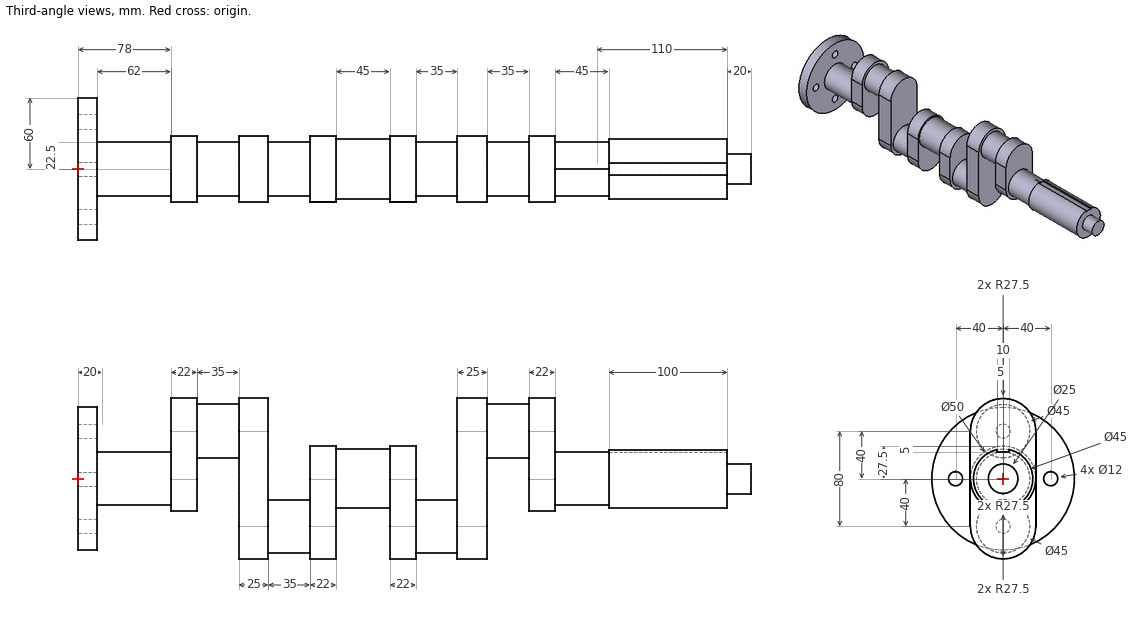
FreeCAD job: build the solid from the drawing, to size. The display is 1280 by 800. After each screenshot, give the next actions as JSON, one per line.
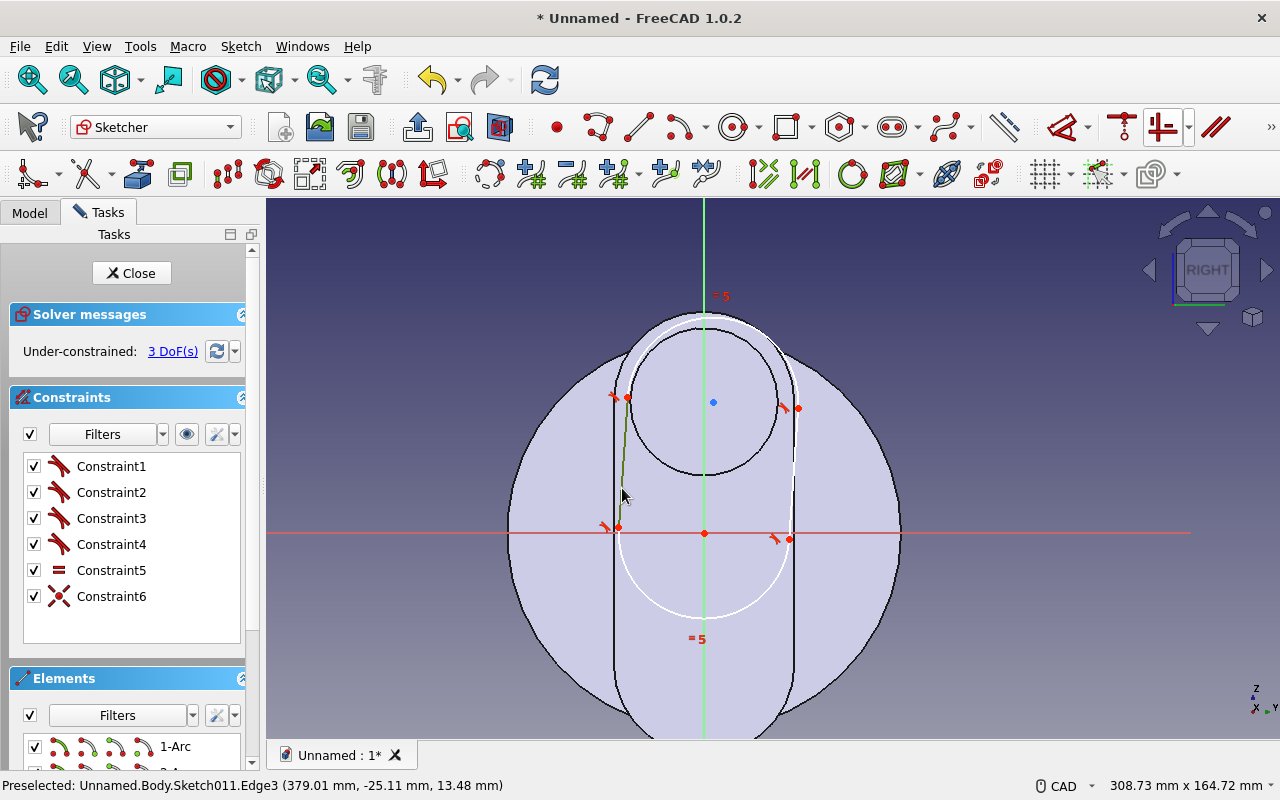
{"action": "key", "text": "v"}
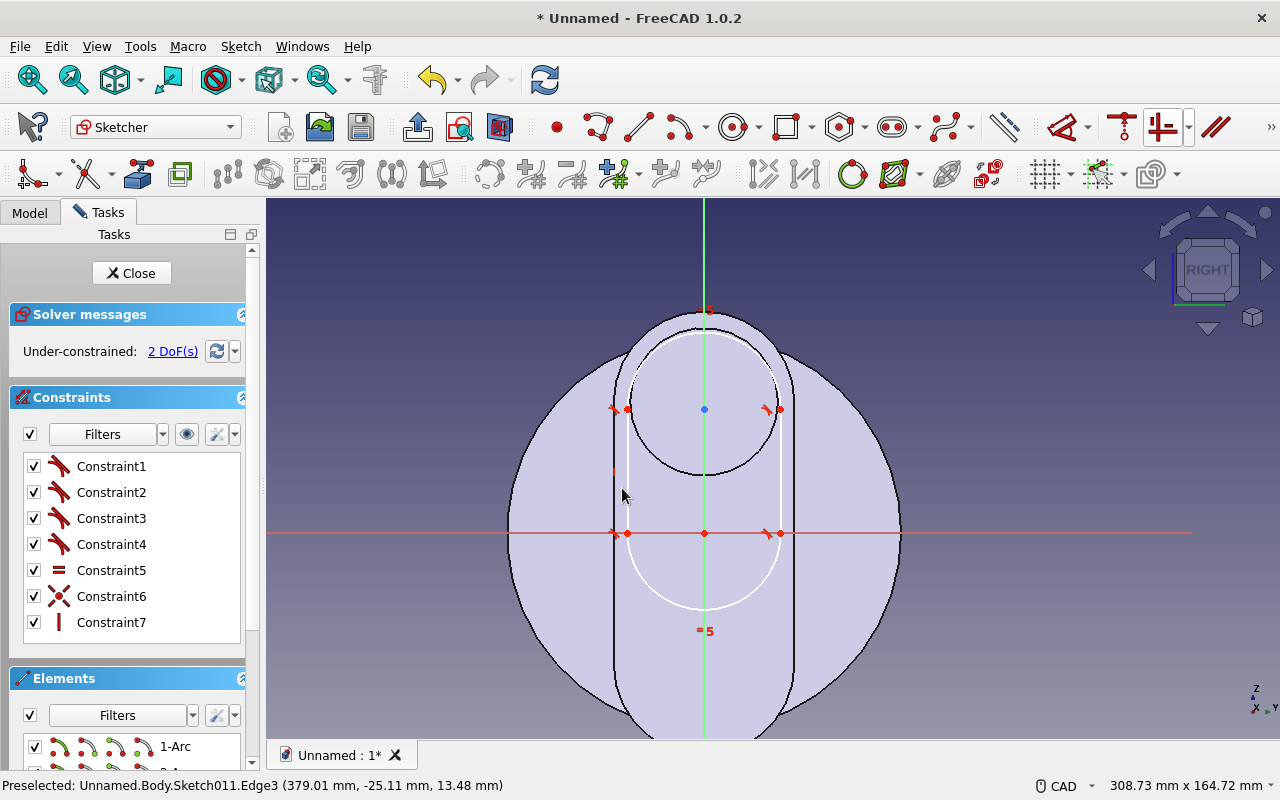
{"action": "key", "text": "d"}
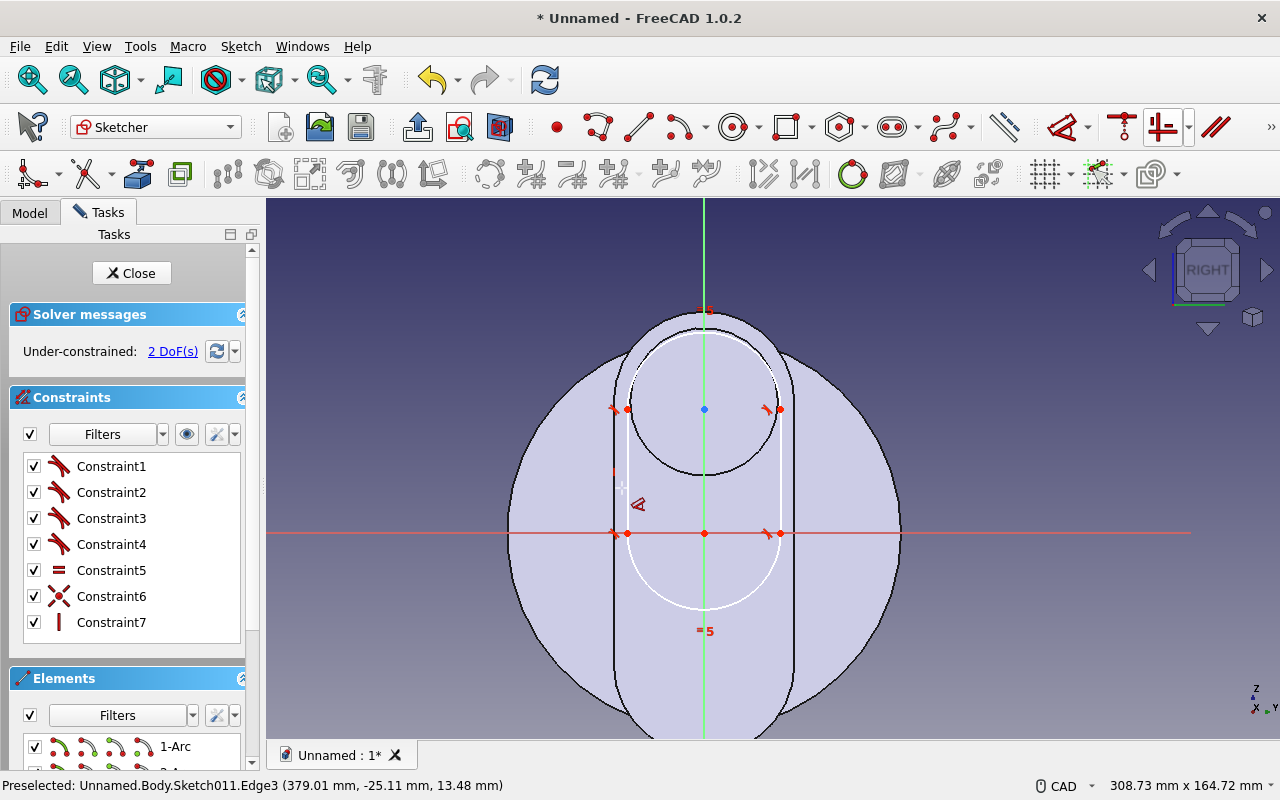
{"action": "left_click", "coordinate": [659, 595]}
{"action": "left_click", "coordinate": [640, 621]}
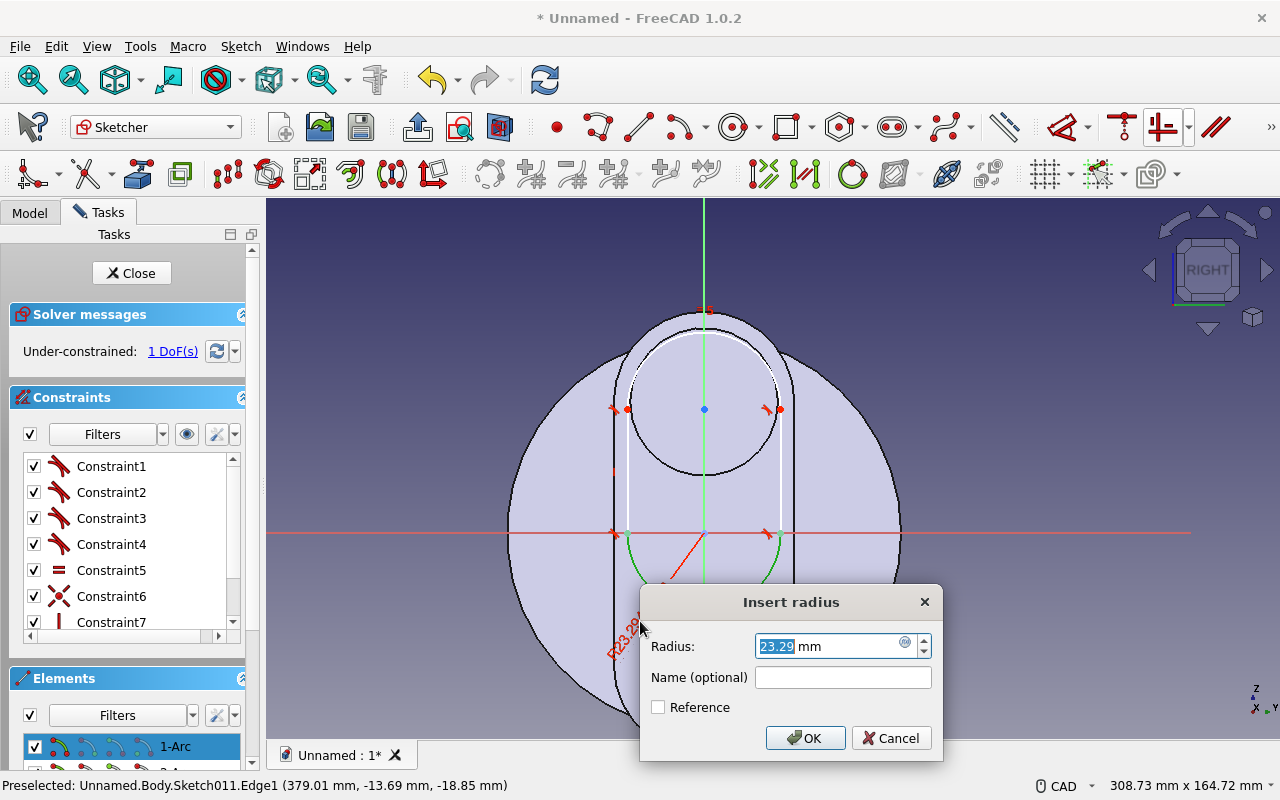
{"action": "type", "text": "27.5"}
{"action": "key", "text": "Return"}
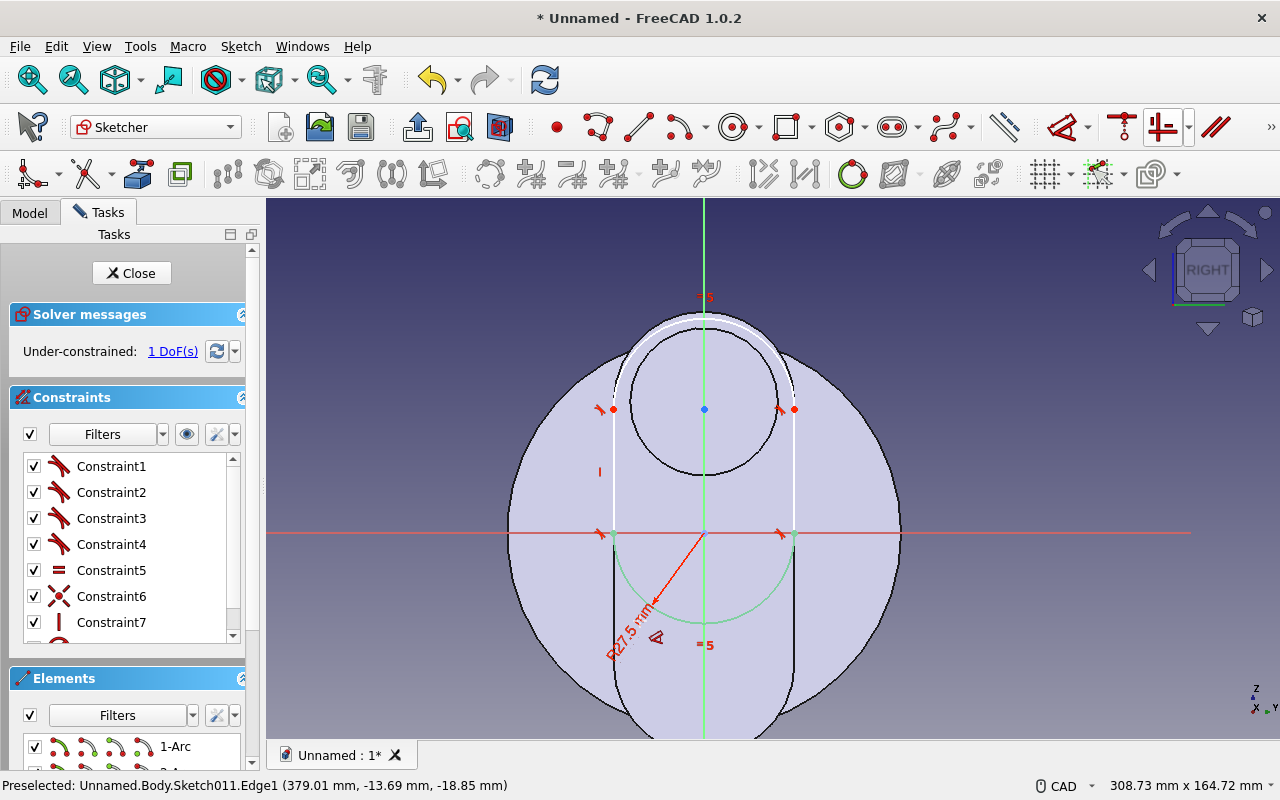
{"action": "left_click", "coordinate": [614, 496]}
{"action": "left_click", "coordinate": [580, 471]}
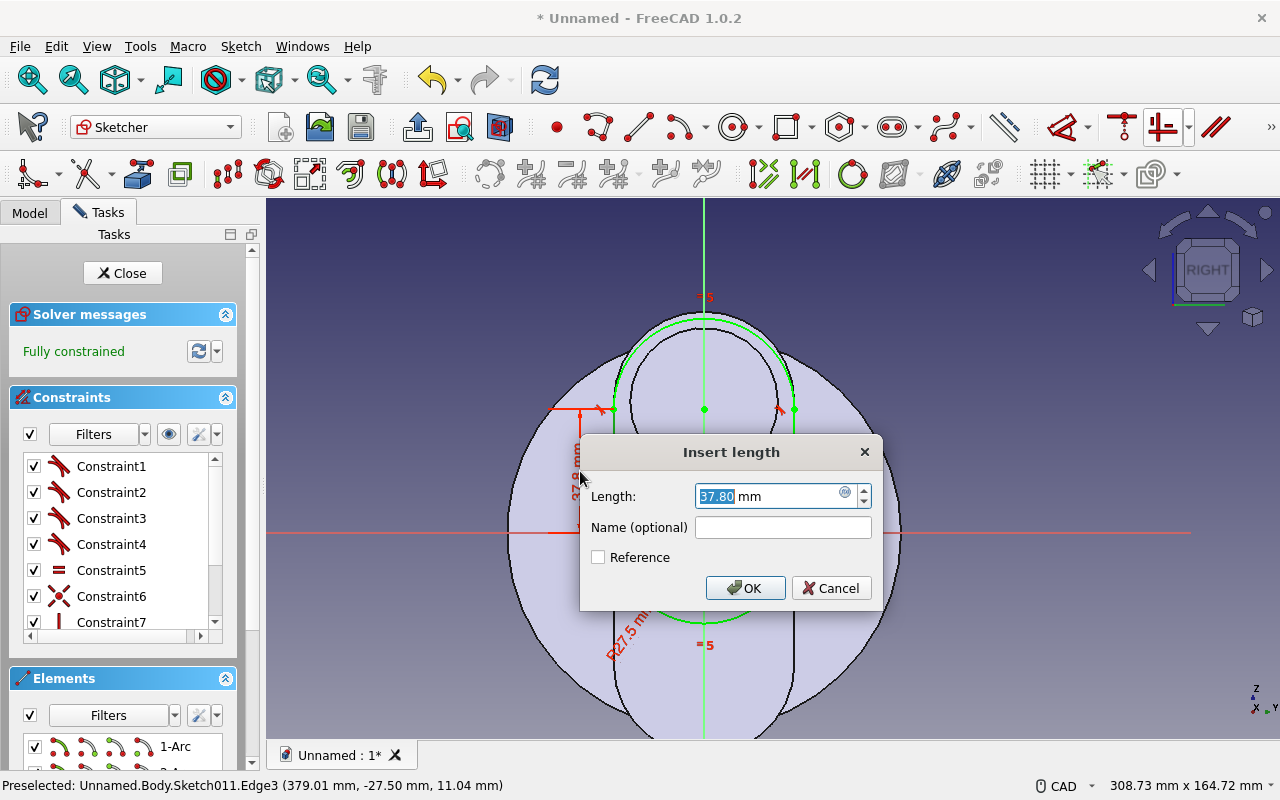
{"action": "type", "text": "40"}
{"action": "key", "text": "Return"}
{"action": "key", "text": "Escape"}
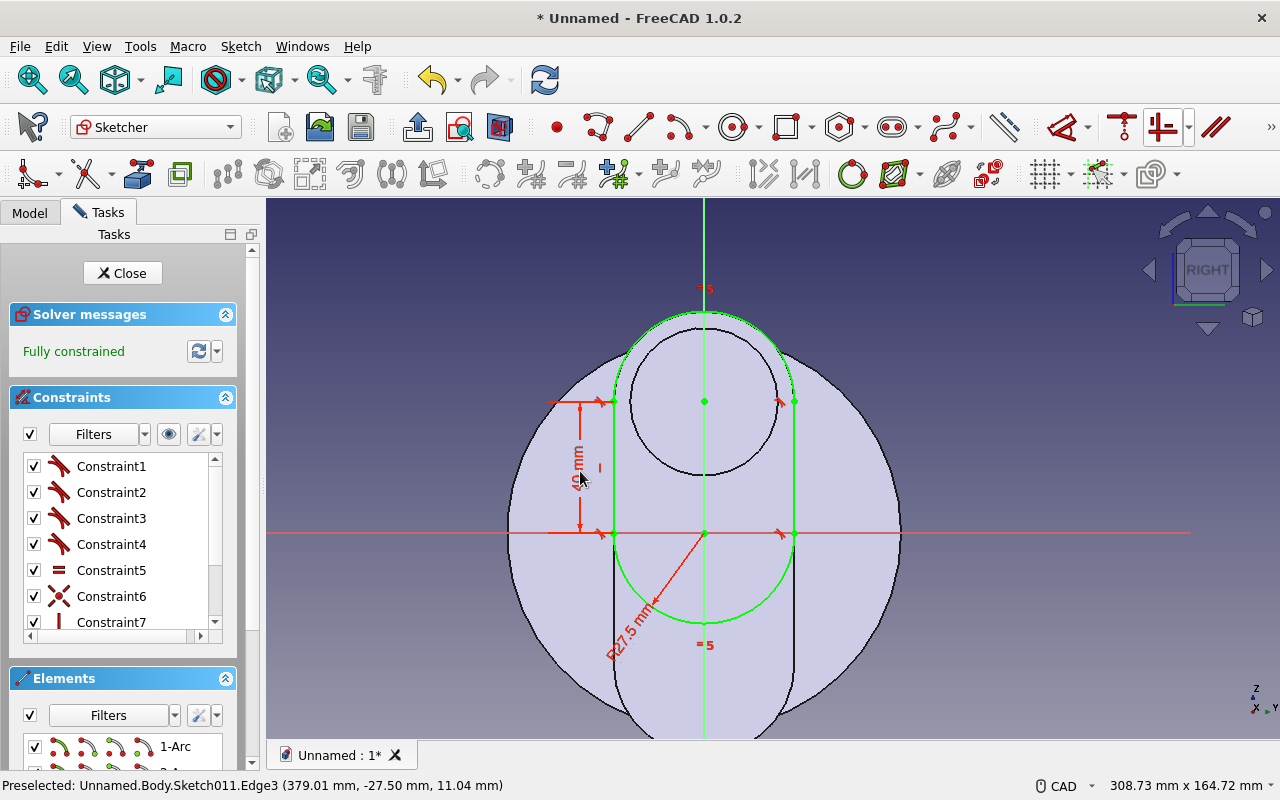
{"action": "left_click", "coordinate": [123, 273]}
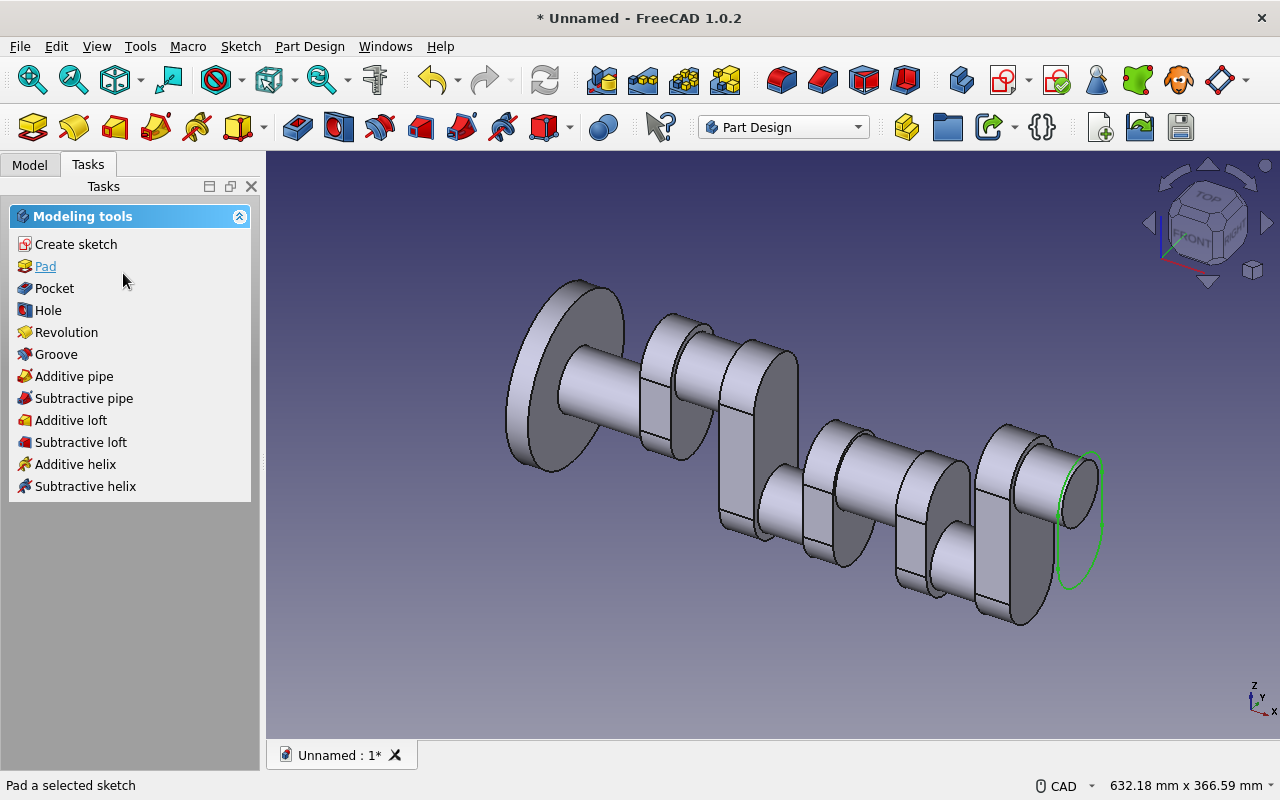
{"action": "left_click", "coordinate": [33, 128]}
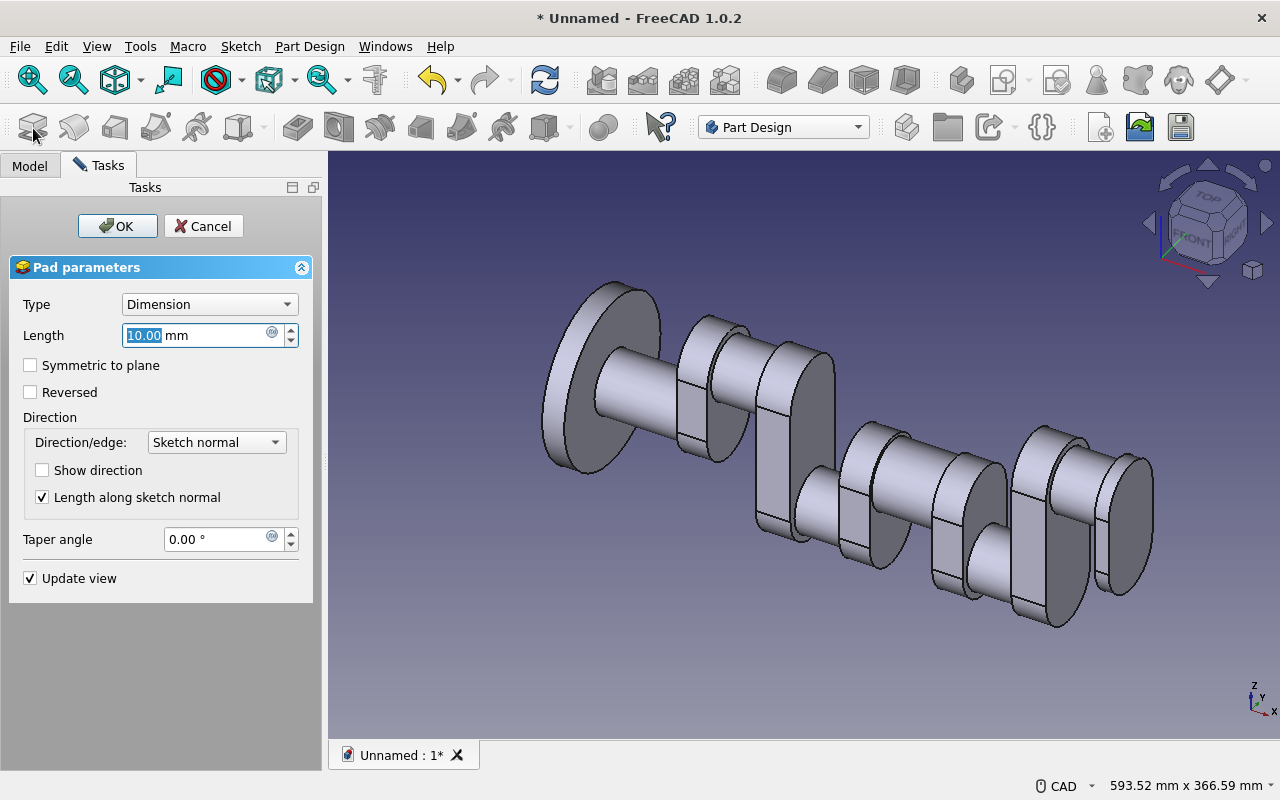
{"action": "type", "text": "22"}
{"action": "key", "text": "Tab"}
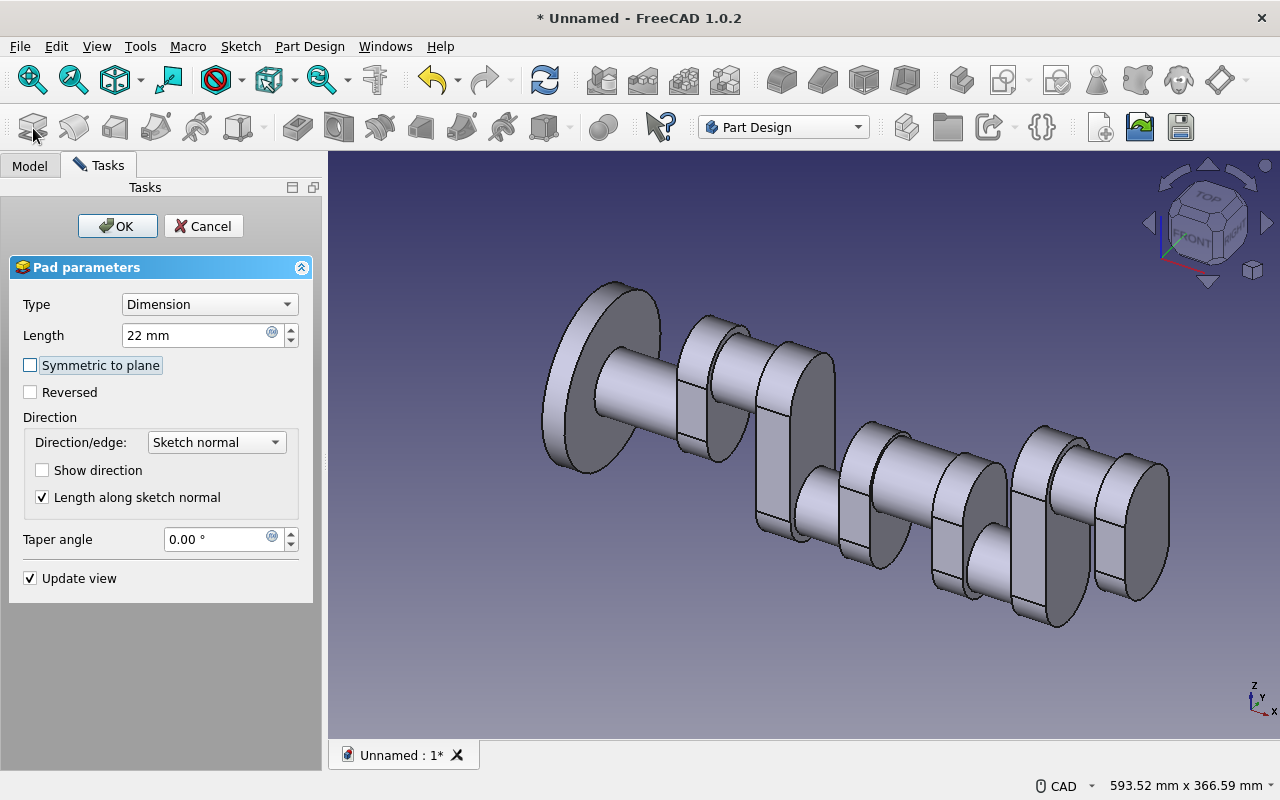
{"action": "left_click", "coordinate": [118, 226]}